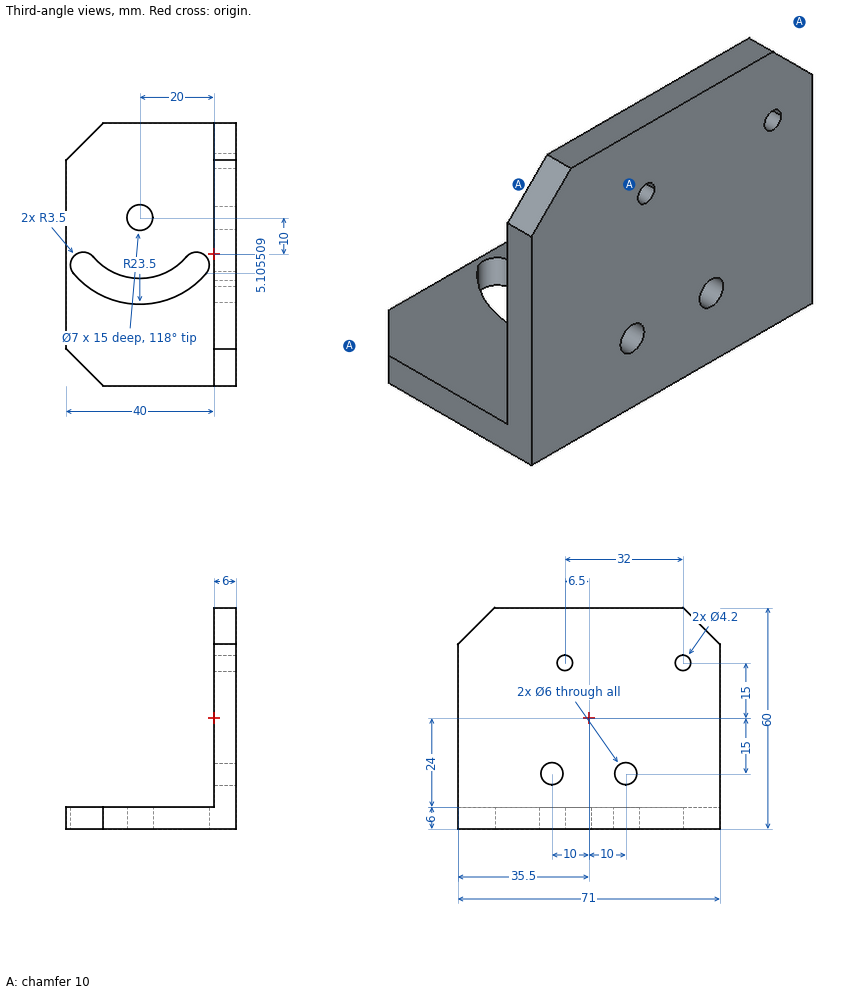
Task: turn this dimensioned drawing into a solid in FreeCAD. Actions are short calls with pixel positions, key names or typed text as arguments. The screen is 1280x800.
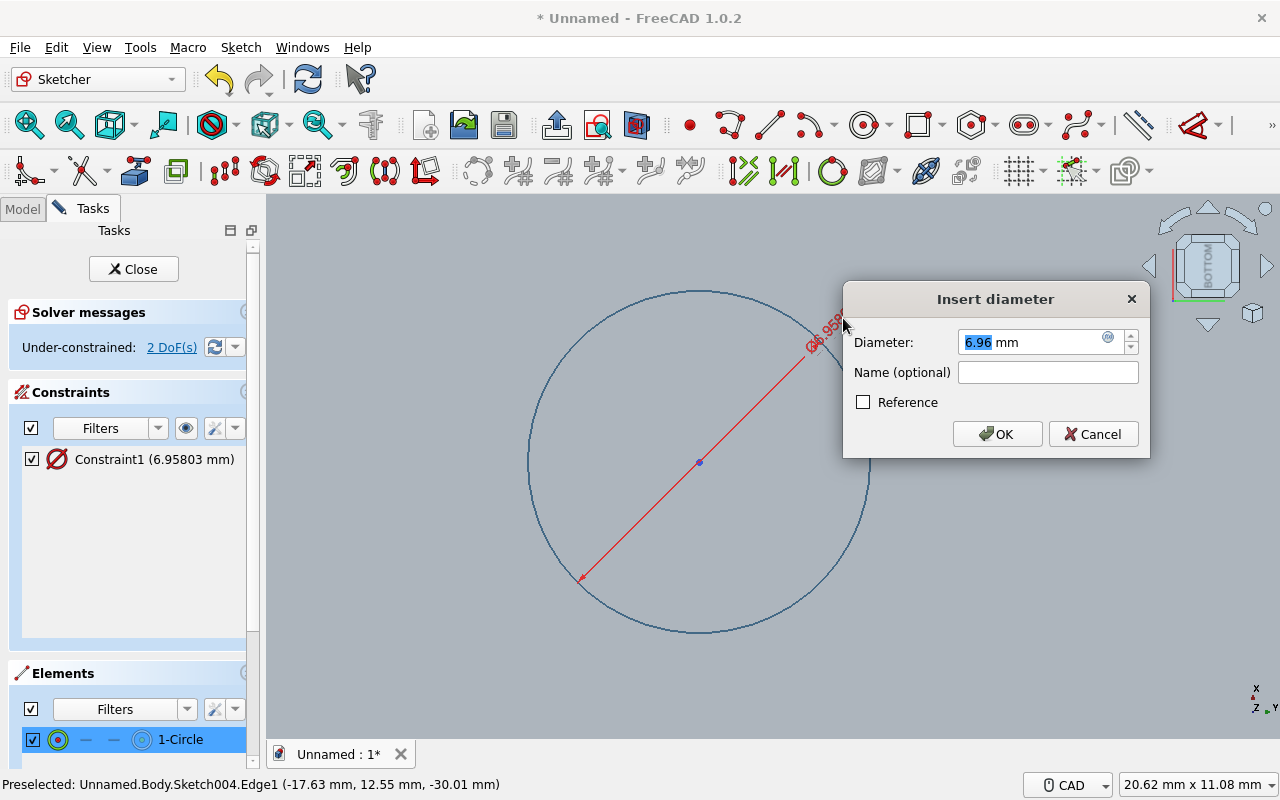
text(7)
key(Return)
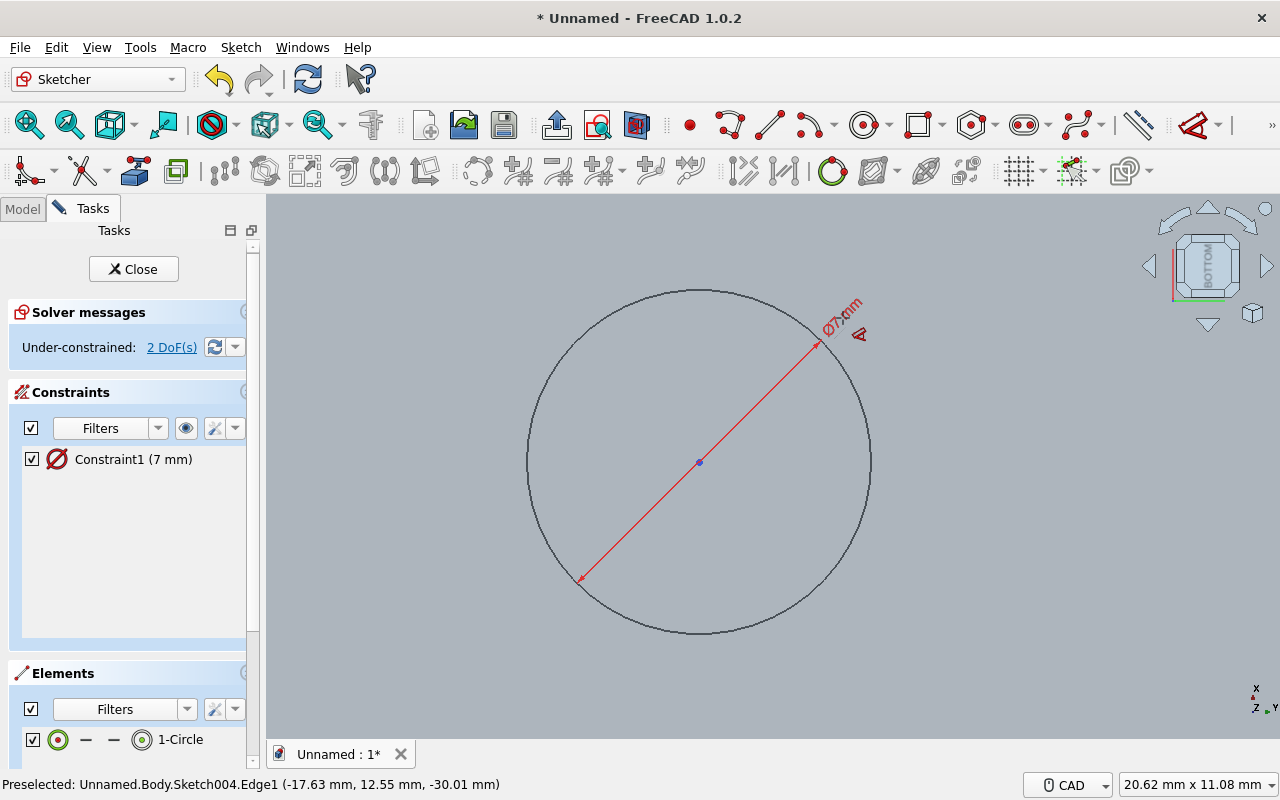
click(699, 462)
click(496, 496)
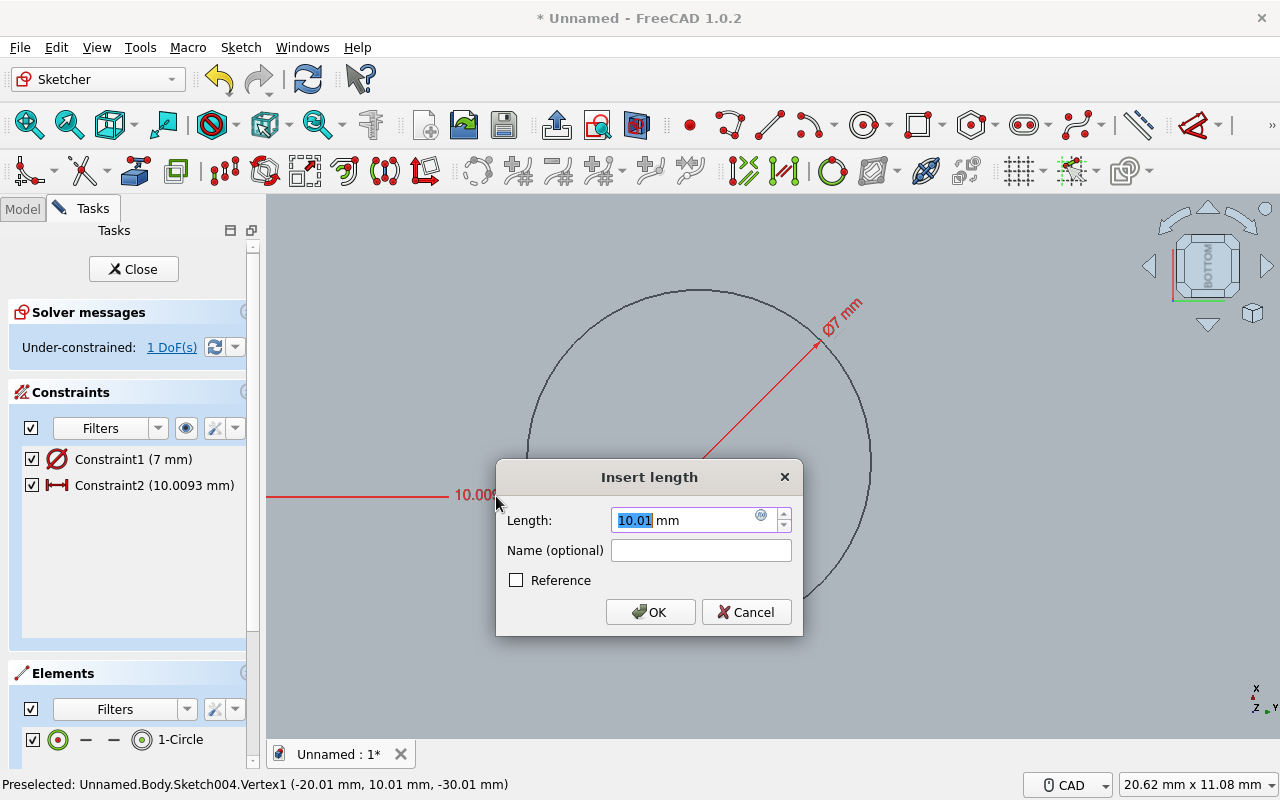
text(10)
key(Return)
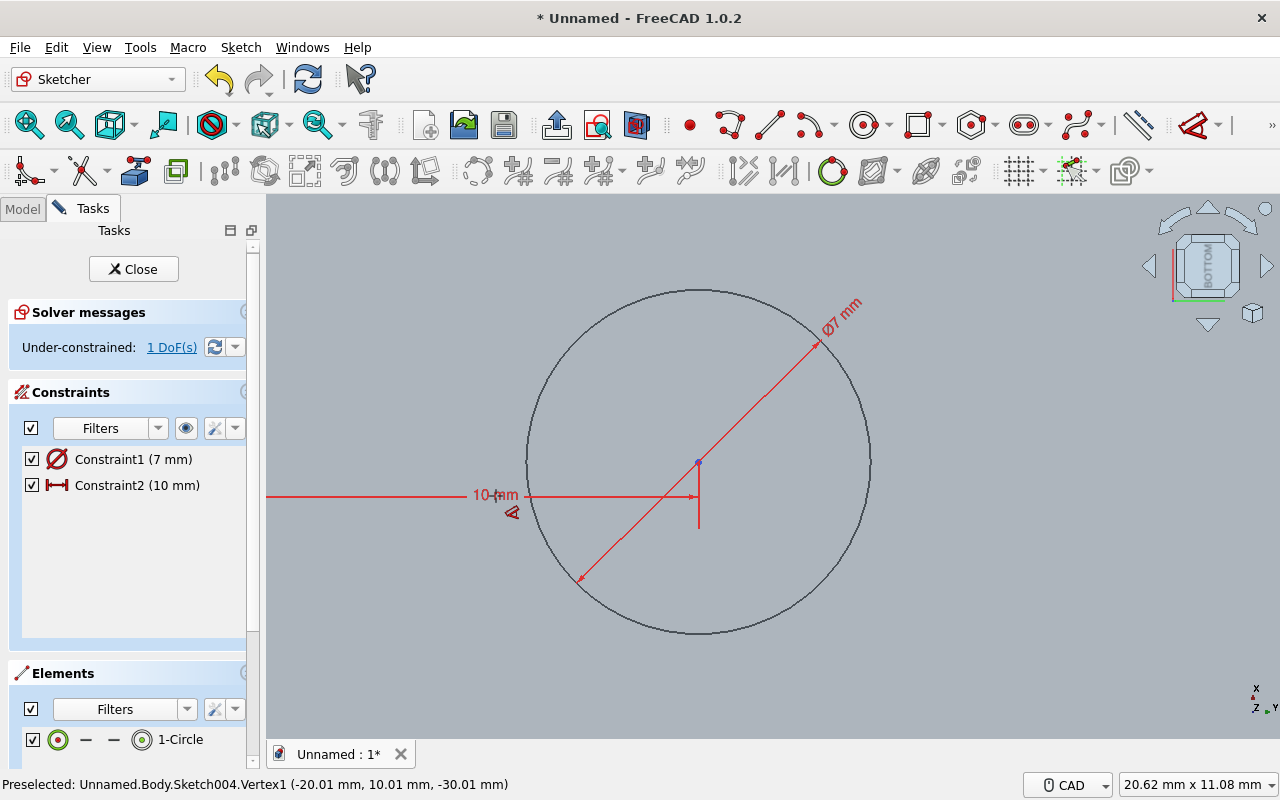
click(699, 462)
click(733, 342)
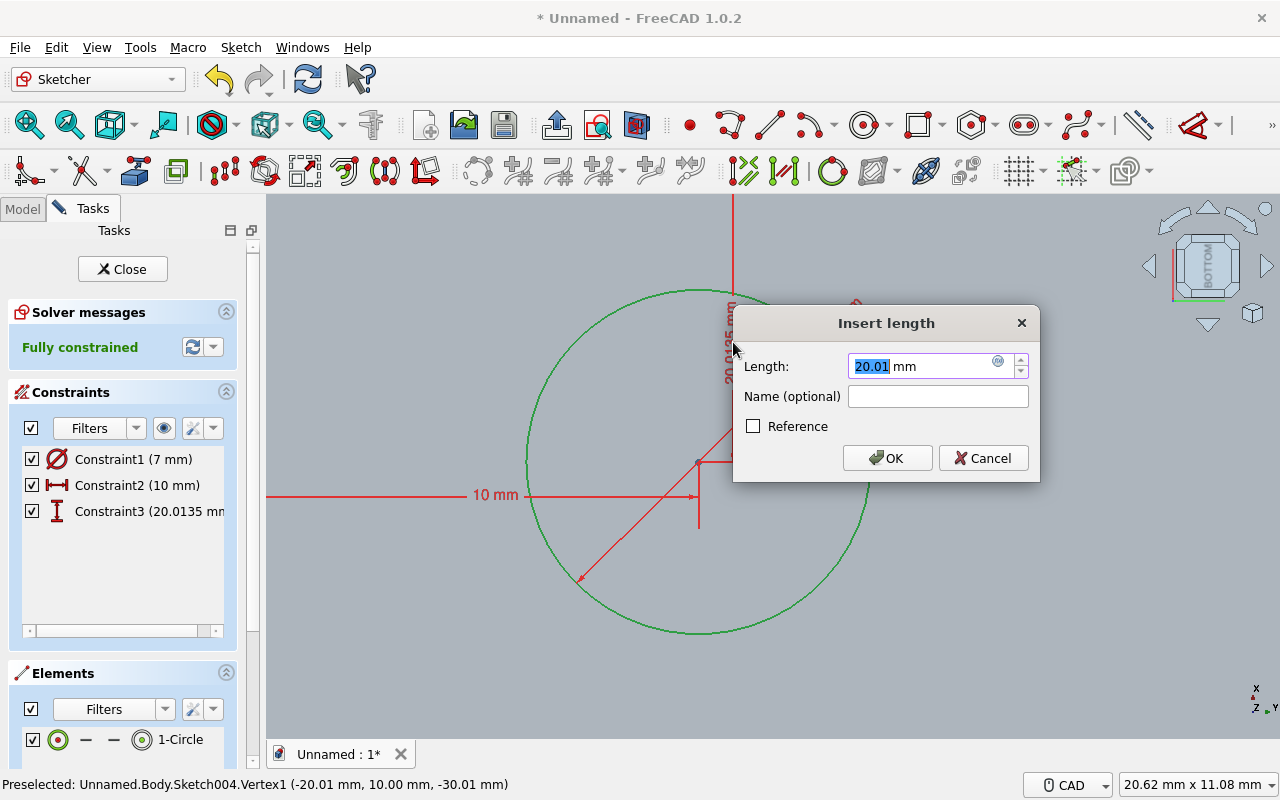
text(20)
key(Return)
key(Escape)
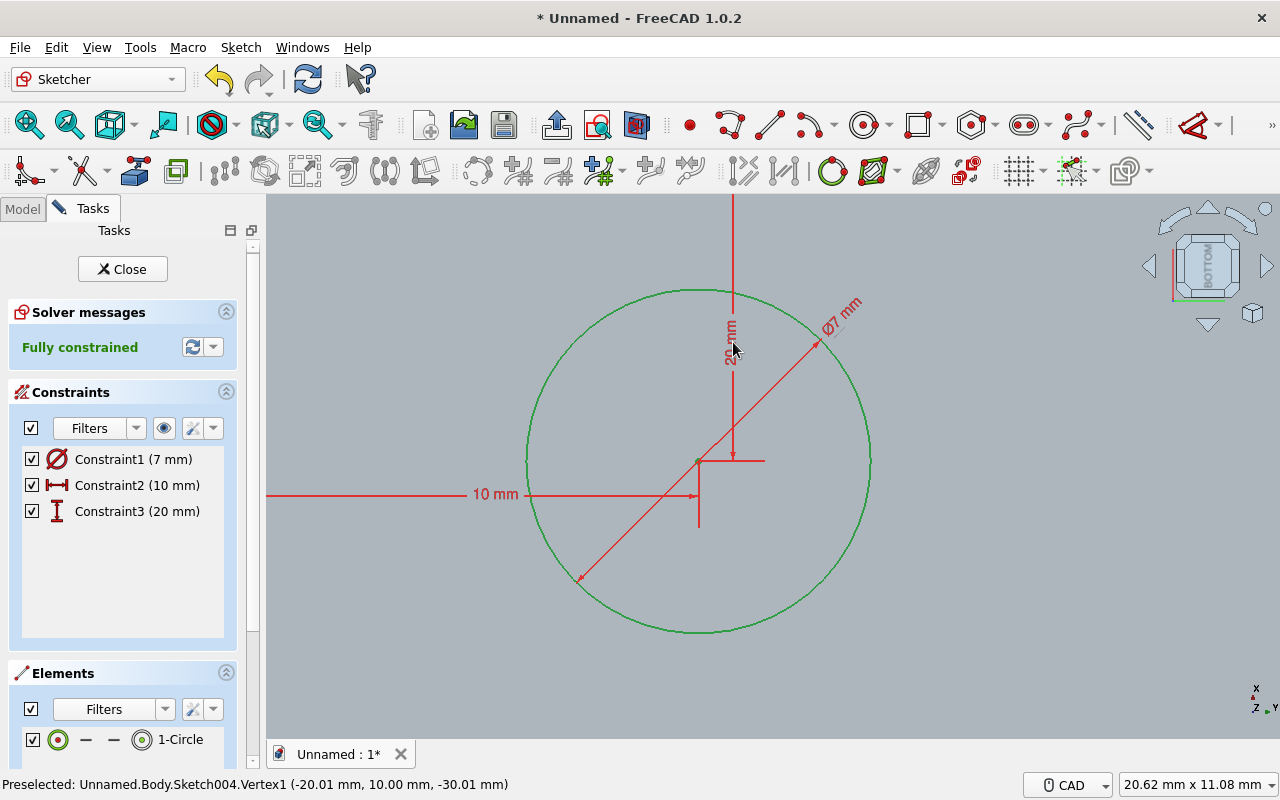
click(123, 269)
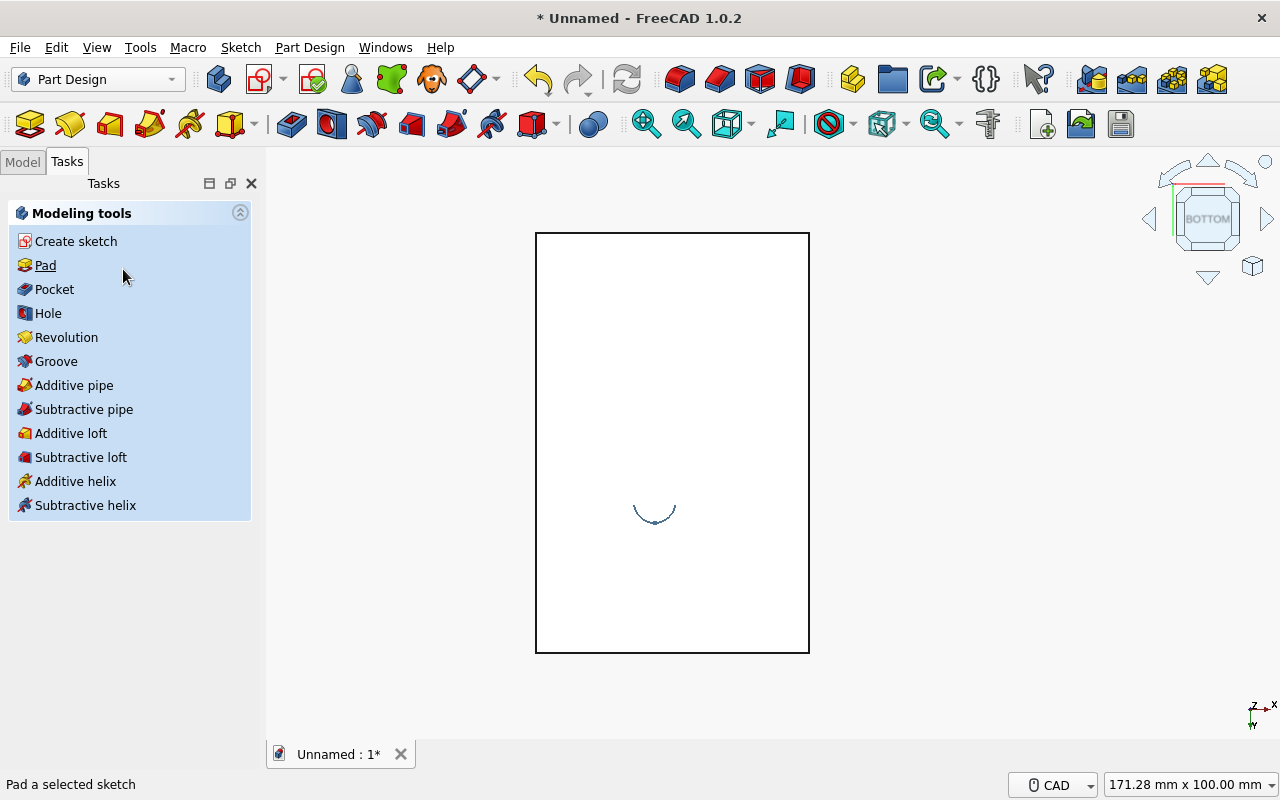
click(332, 124)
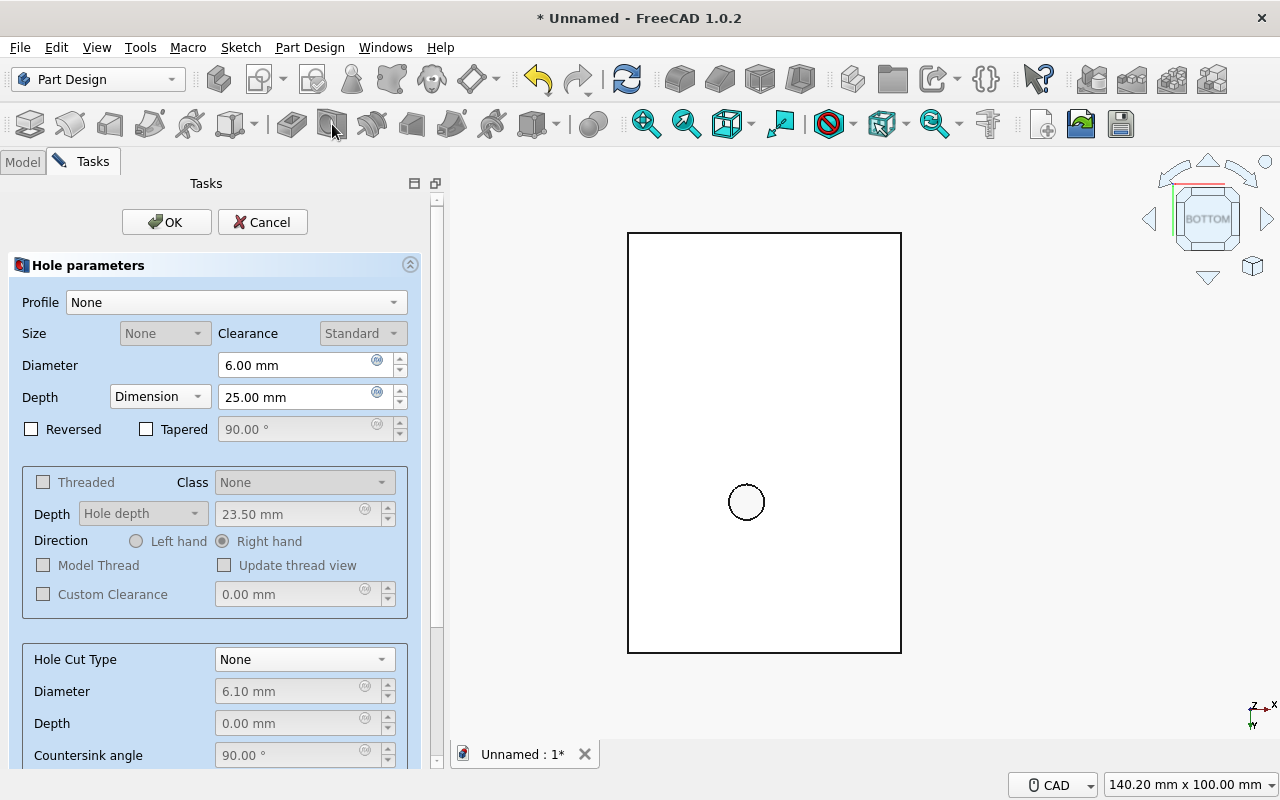
triple_click(305, 365)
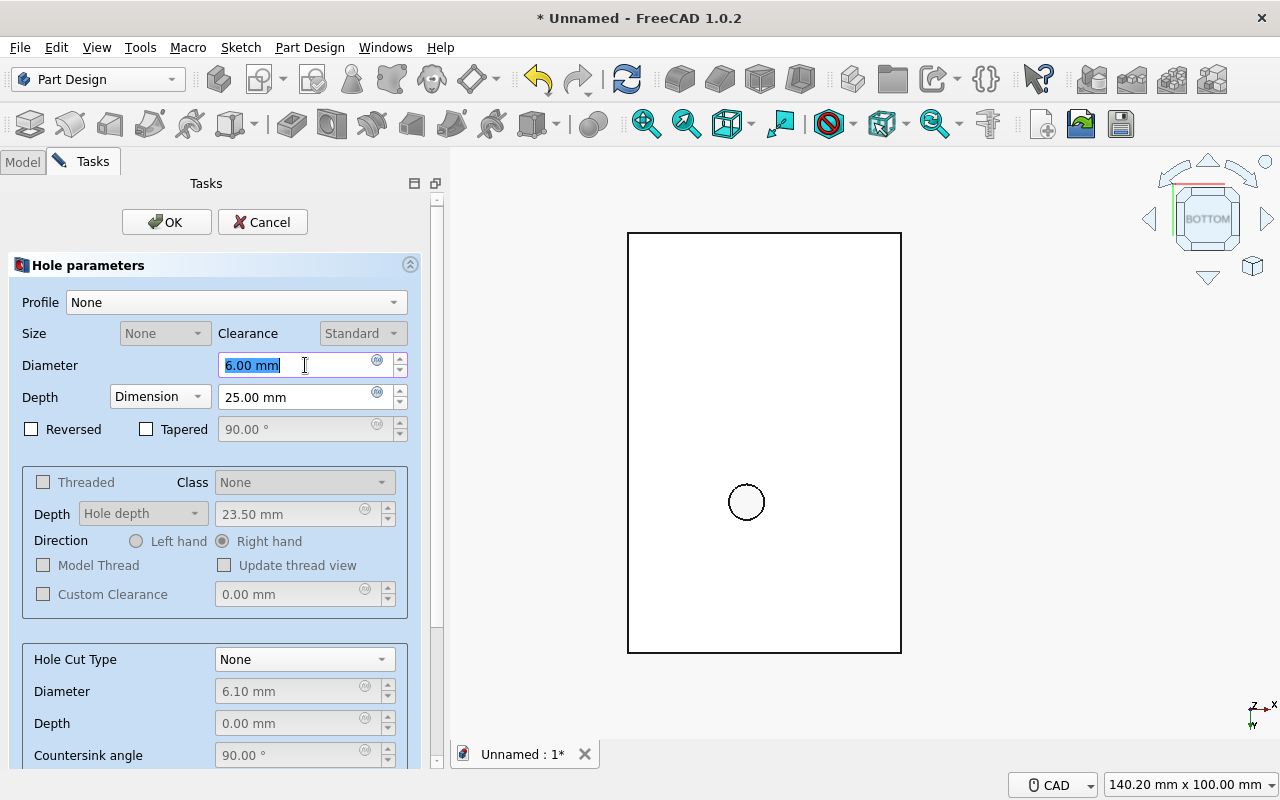
text(7)
key(Tab)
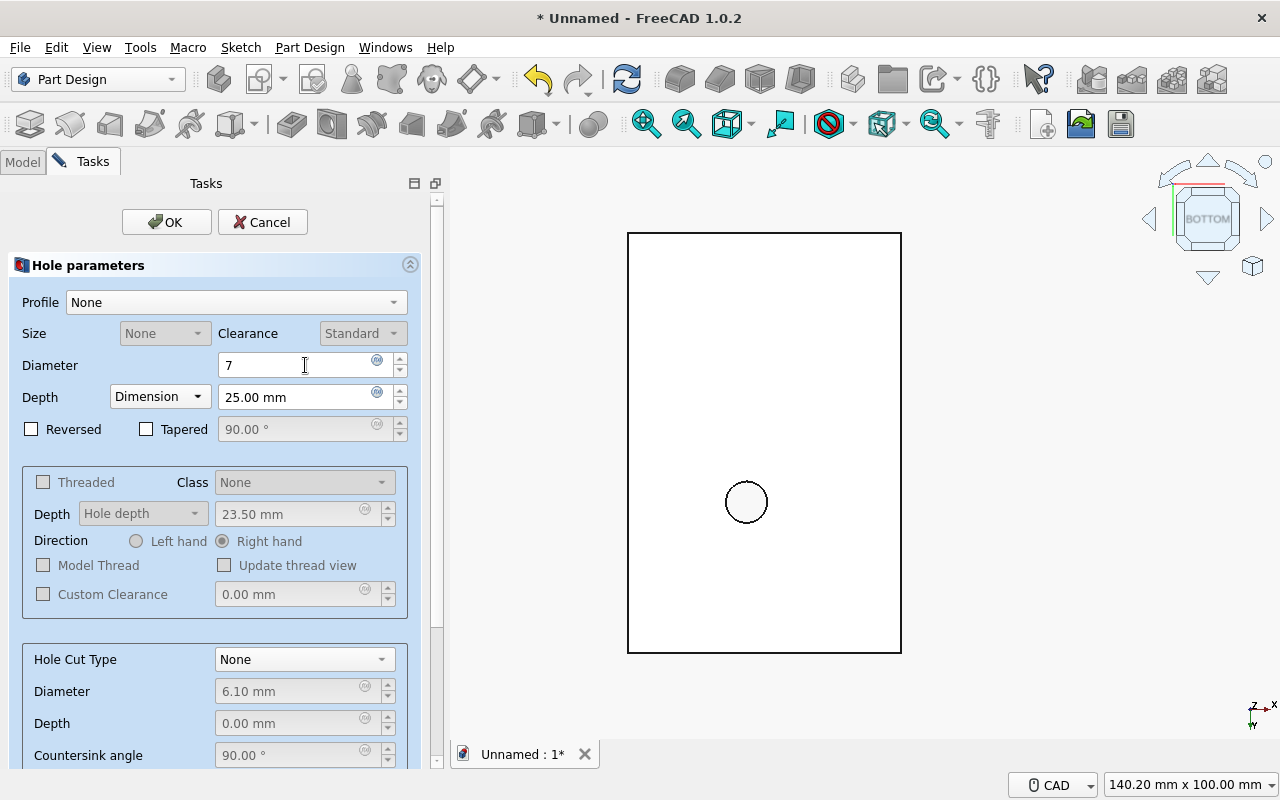
triple_click(305, 397)